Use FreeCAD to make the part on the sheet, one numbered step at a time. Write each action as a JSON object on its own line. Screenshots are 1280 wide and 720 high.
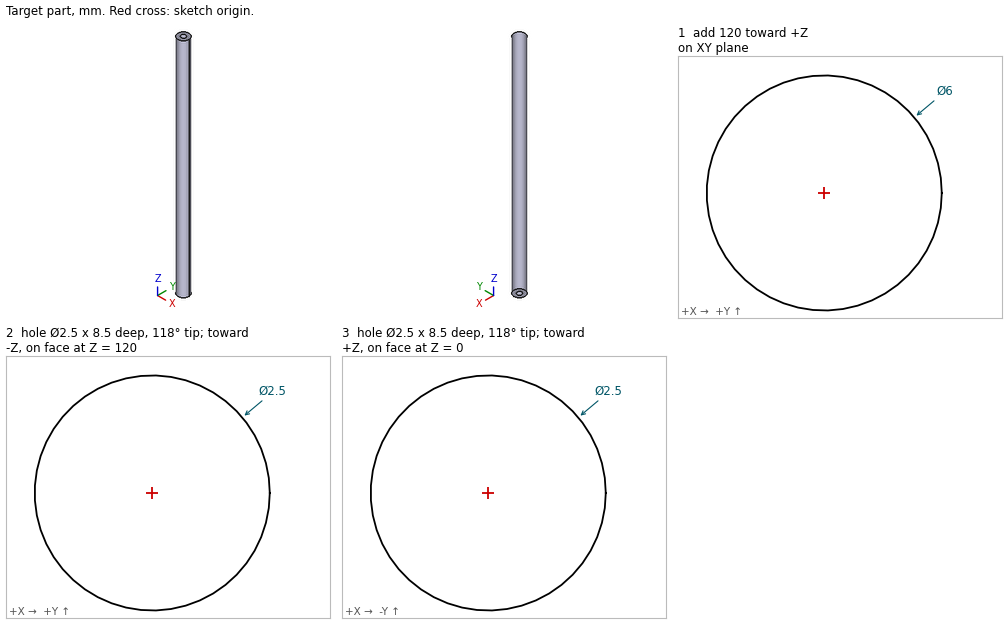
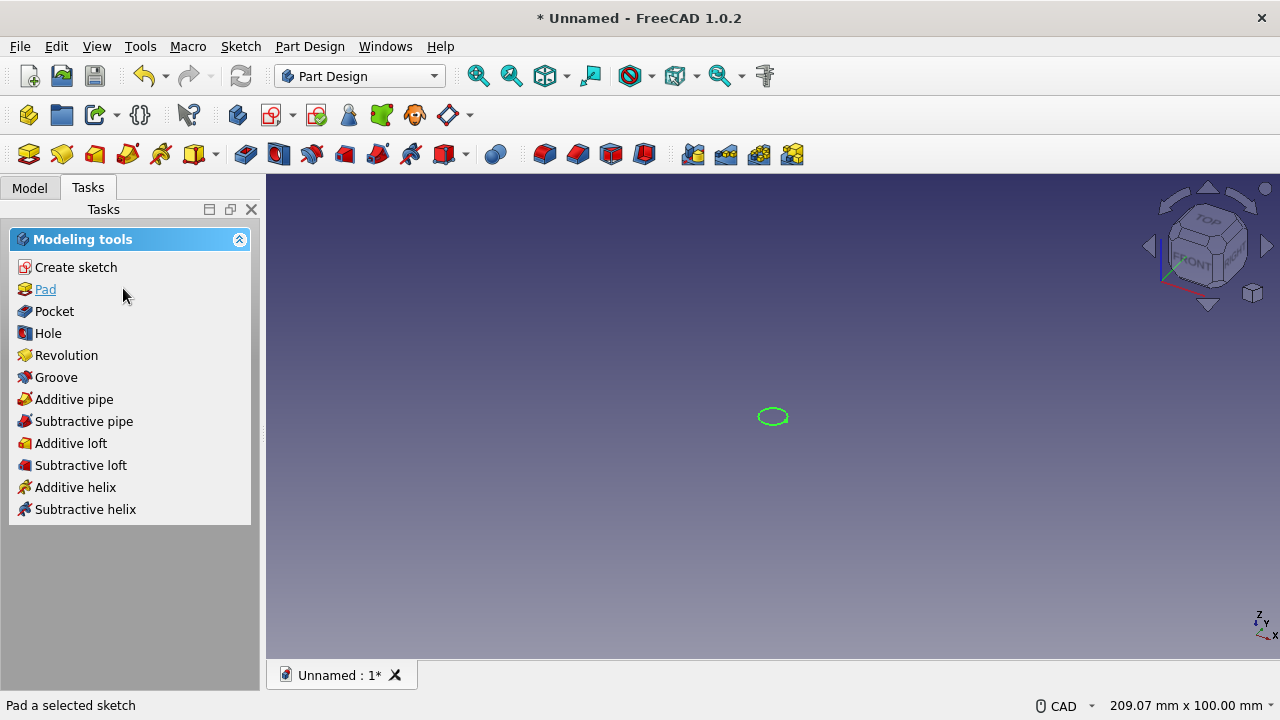
{"action": "left_click", "coordinate": [29, 154]}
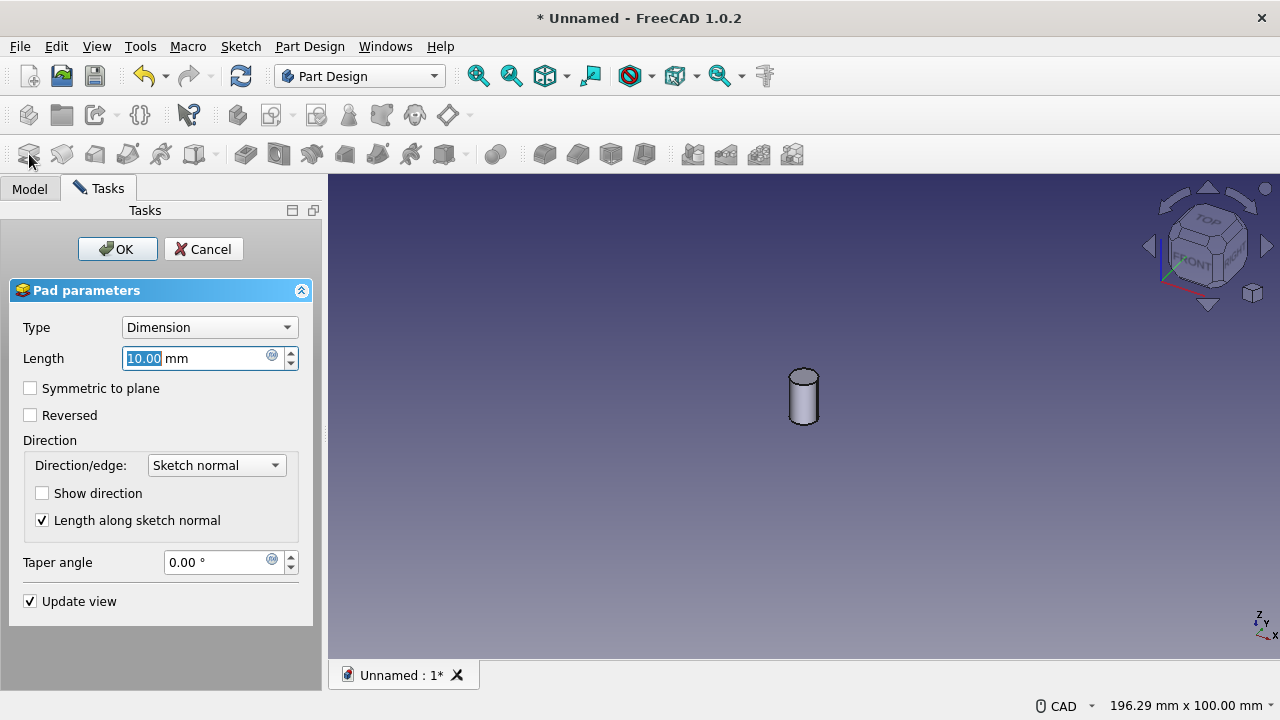
{"action": "type", "text": "120"}
{"action": "key", "text": "Tab"}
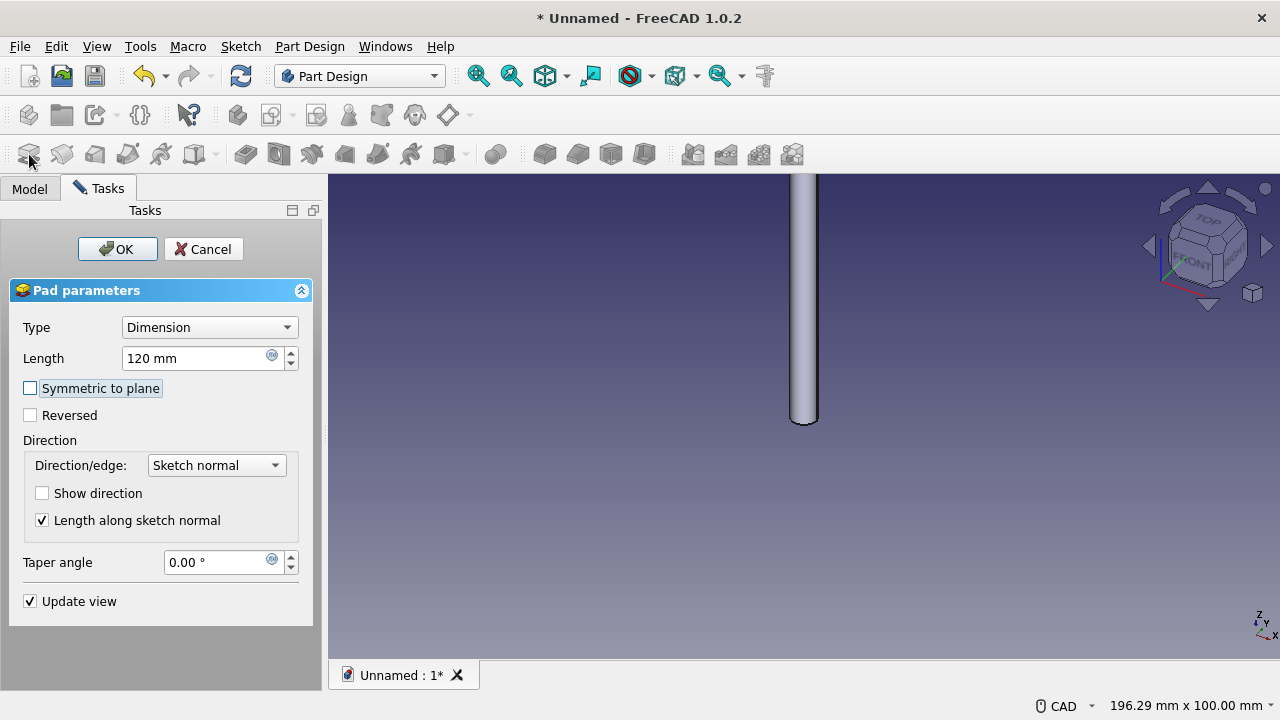
{"action": "left_click", "coordinate": [118, 249]}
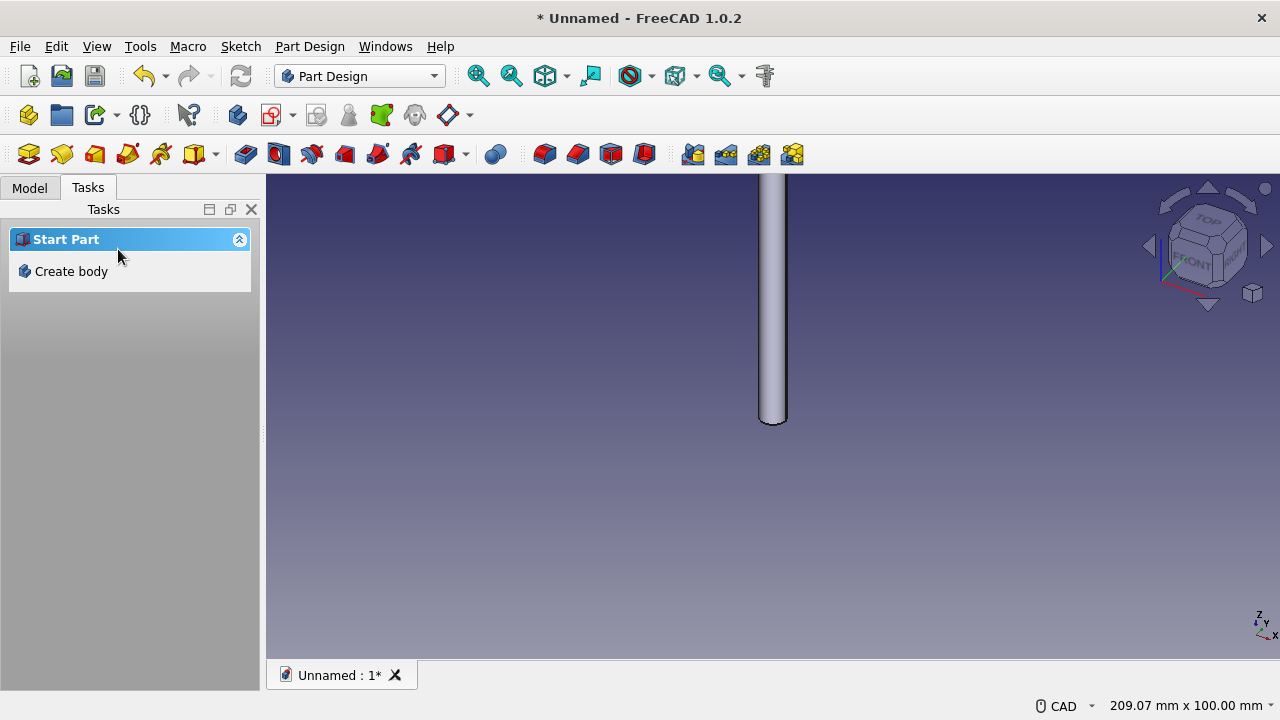
{"action": "key", "text": "v f"}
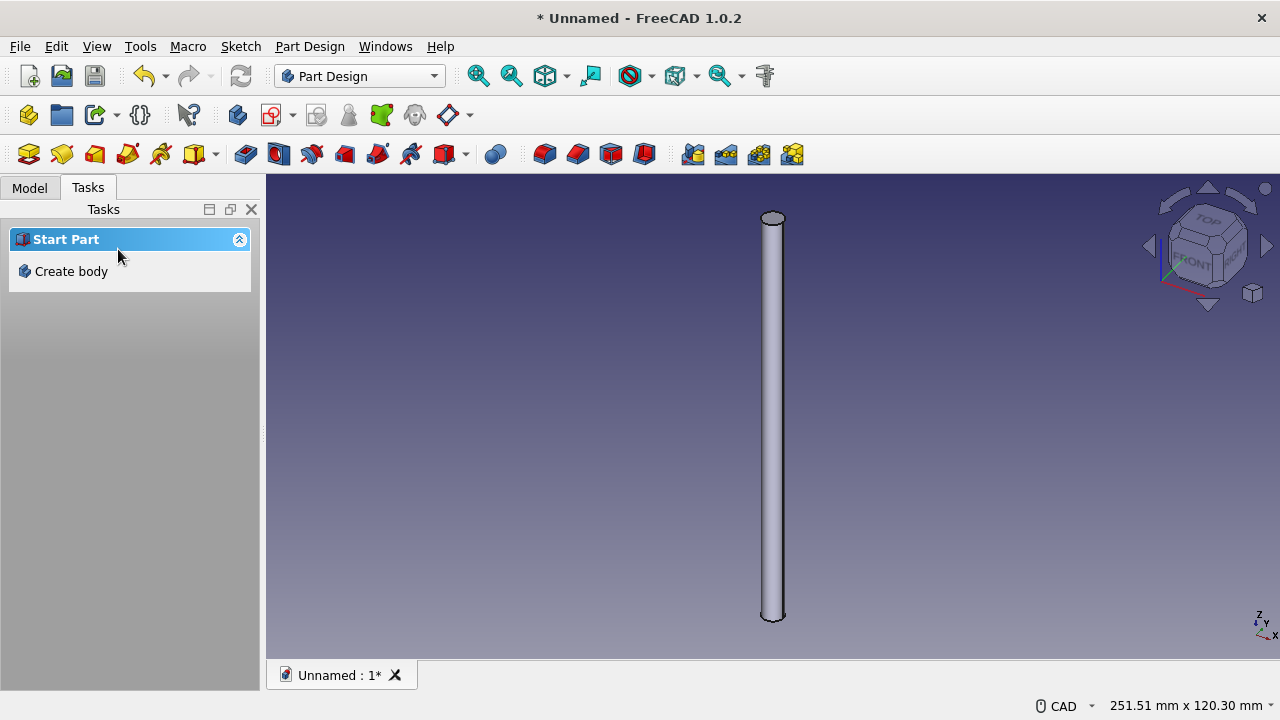
{"action": "left_click", "coordinate": [772, 215]}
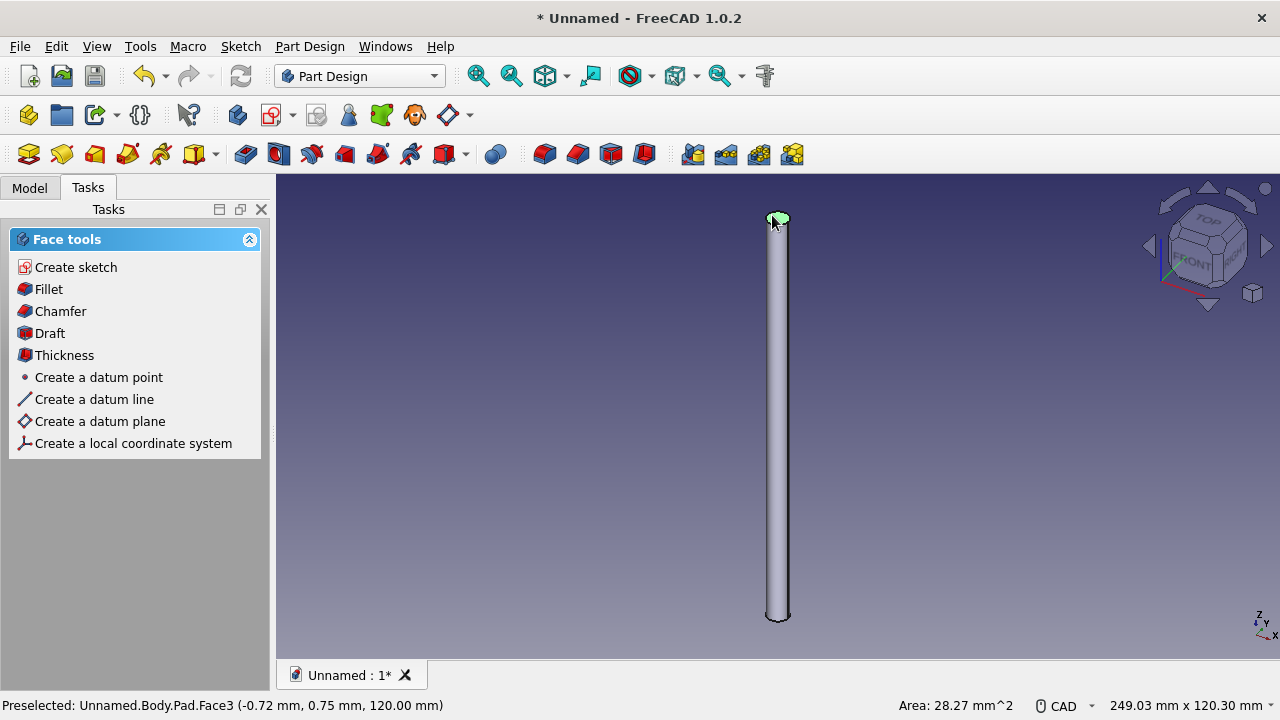
{"action": "left_click", "coordinate": [270, 116]}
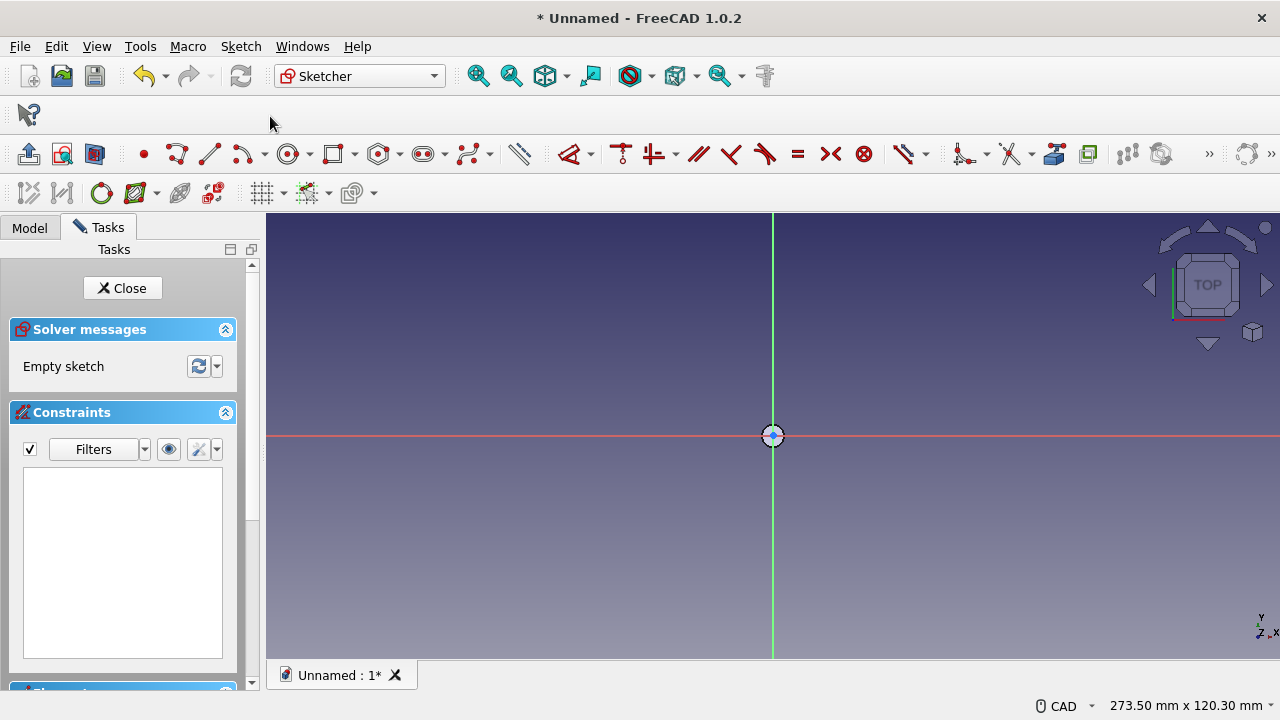
{"action": "scroll", "coordinate": [777, 436], "scroll_direction": "up", "scroll_amount": 15}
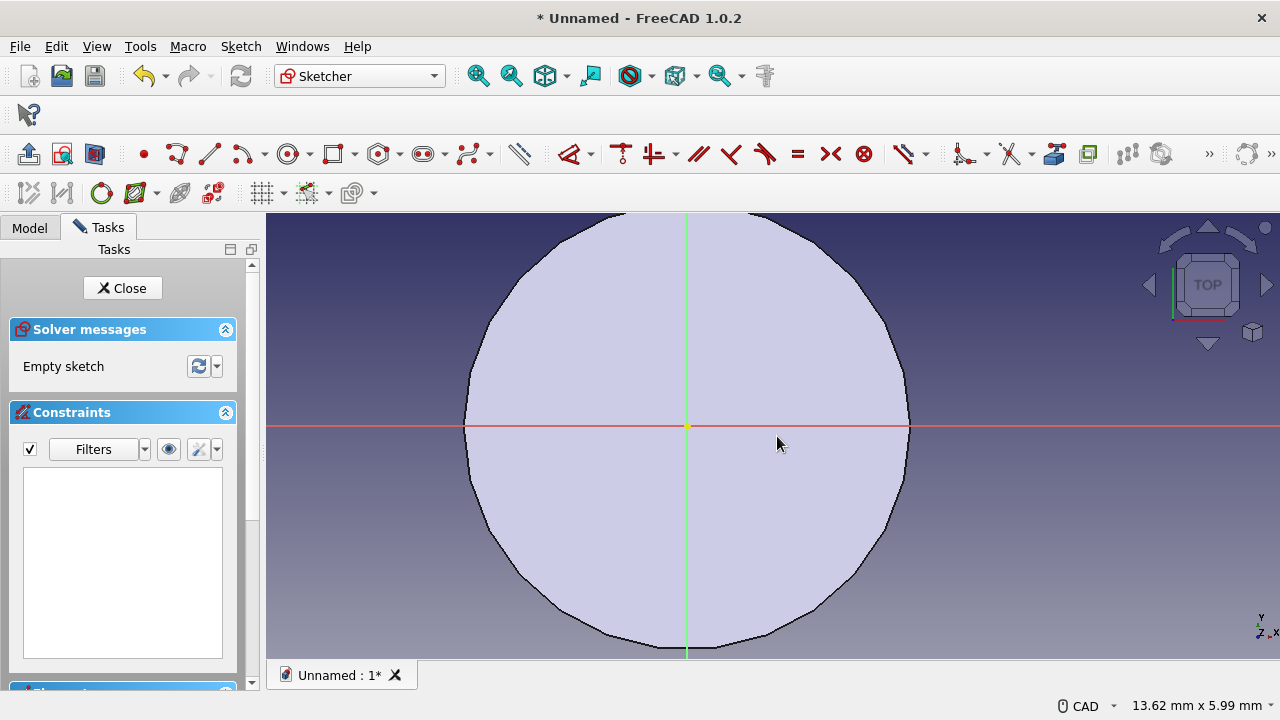
{"action": "scroll", "coordinate": [652, 407], "scroll_direction": "up", "scroll_amount": 2}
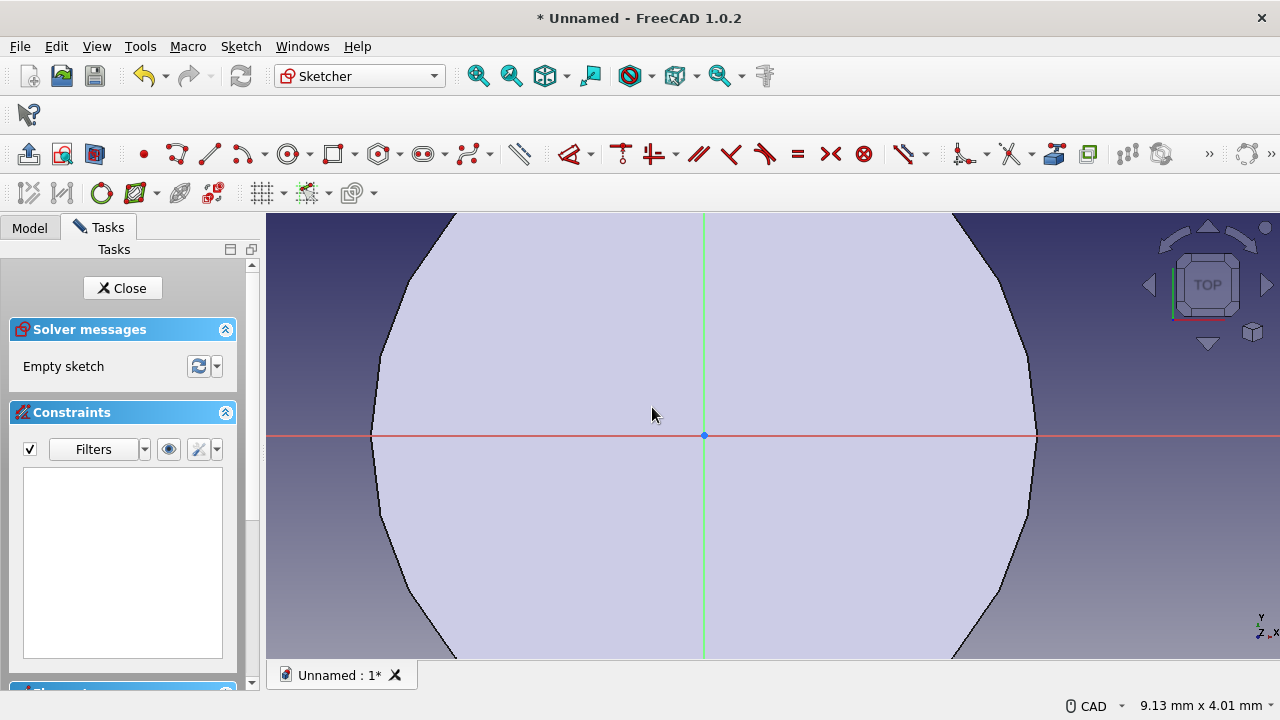
{"action": "key", "text": "g c"}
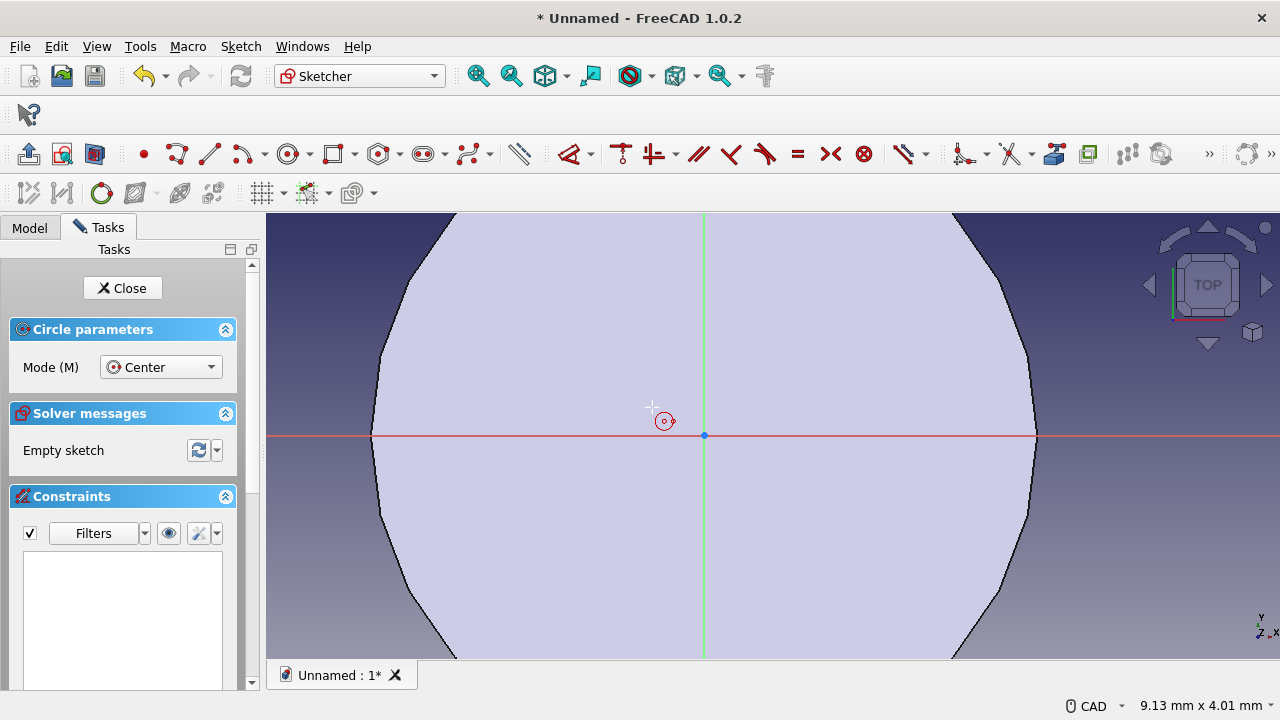
{"action": "left_click", "coordinate": [704, 436]}
{"action": "left_click", "coordinate": [802, 338]}
{"action": "key", "text": "Escape"}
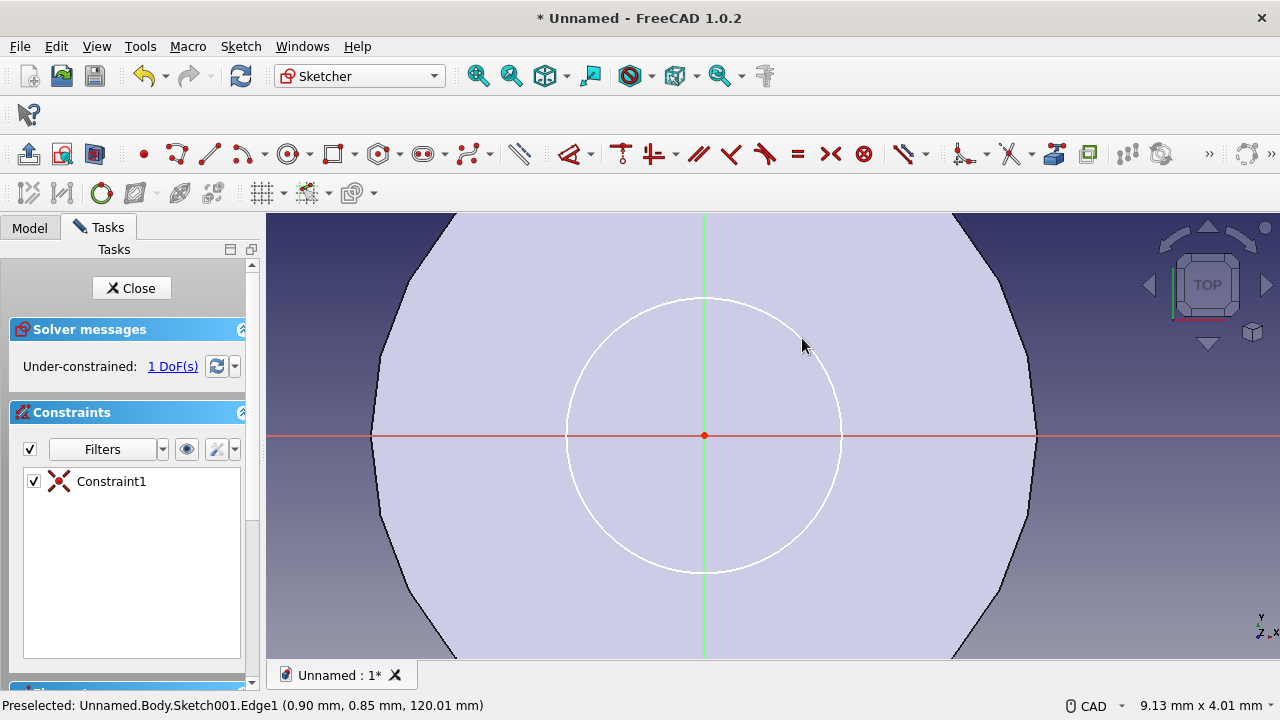
{"action": "left_click", "coordinate": [568, 154]}